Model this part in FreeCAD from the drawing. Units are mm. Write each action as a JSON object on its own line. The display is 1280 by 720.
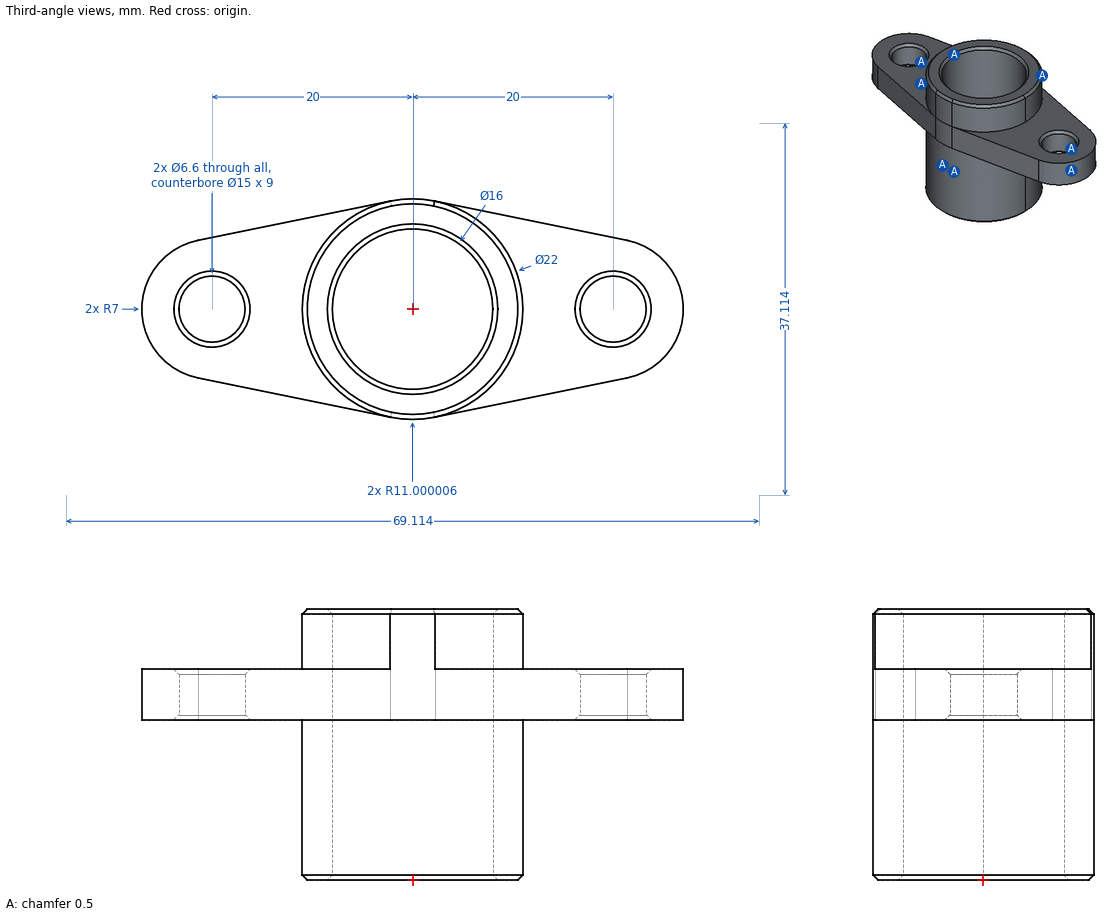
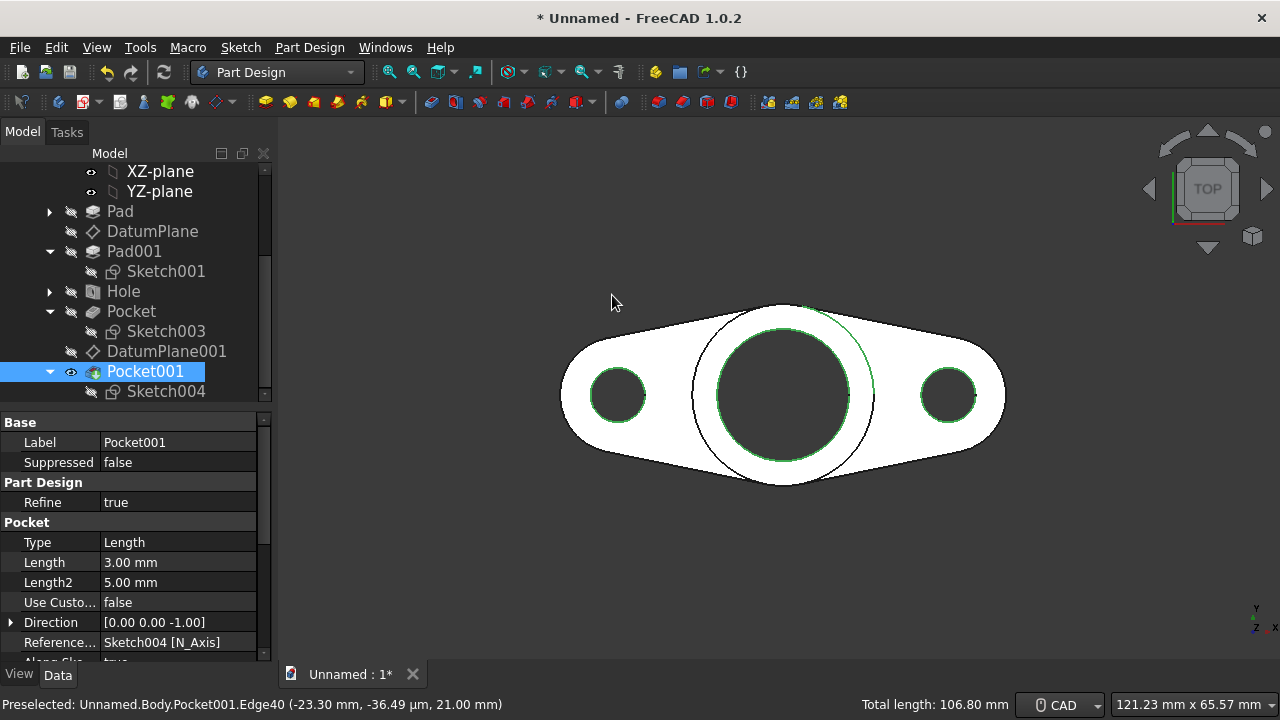
{"action": "left_click", "coordinate": [390, 72]}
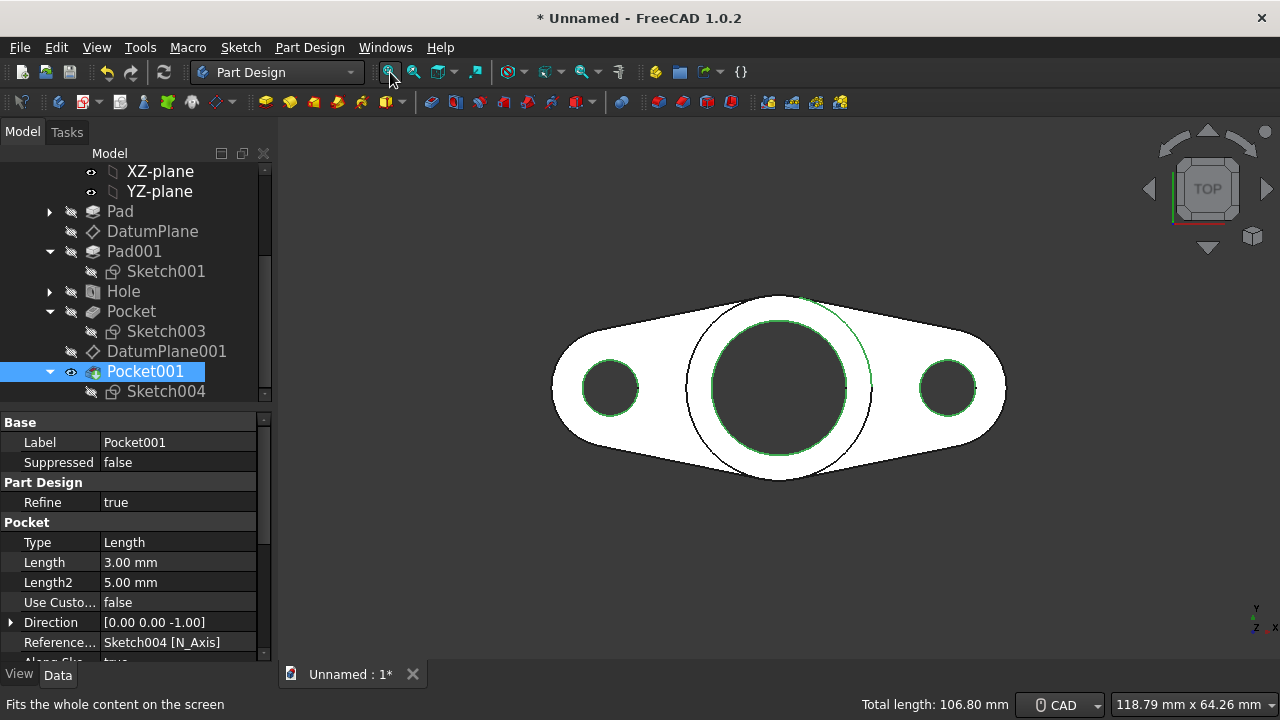
{"action": "key", "text": "1"}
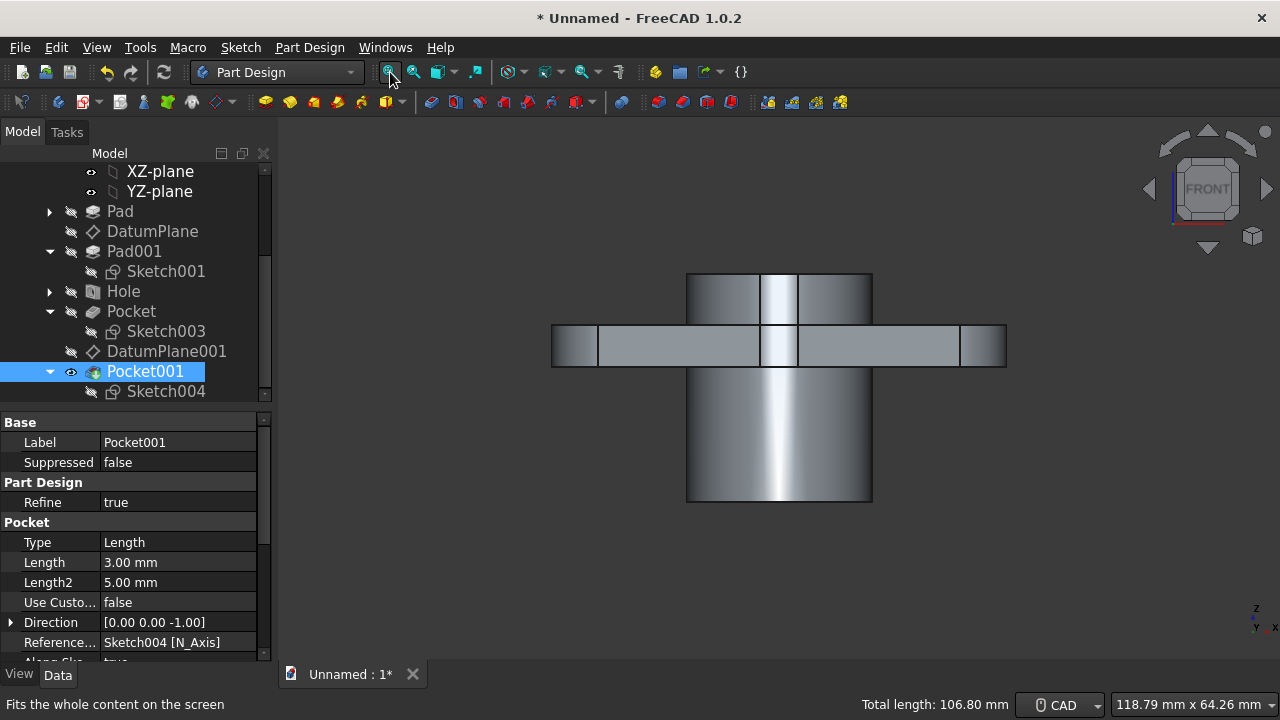
{"action": "left_click", "coordinate": [847, 501], "text": "ctrl"}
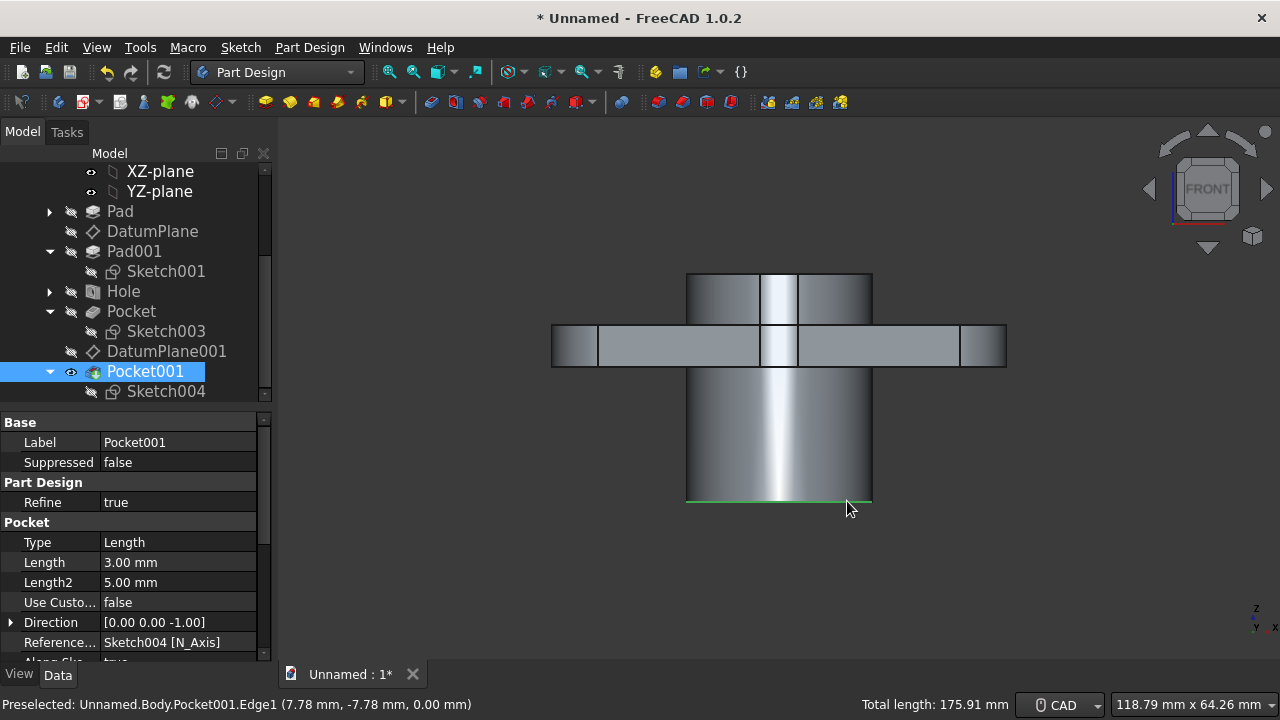
{"action": "key", "text": "3"}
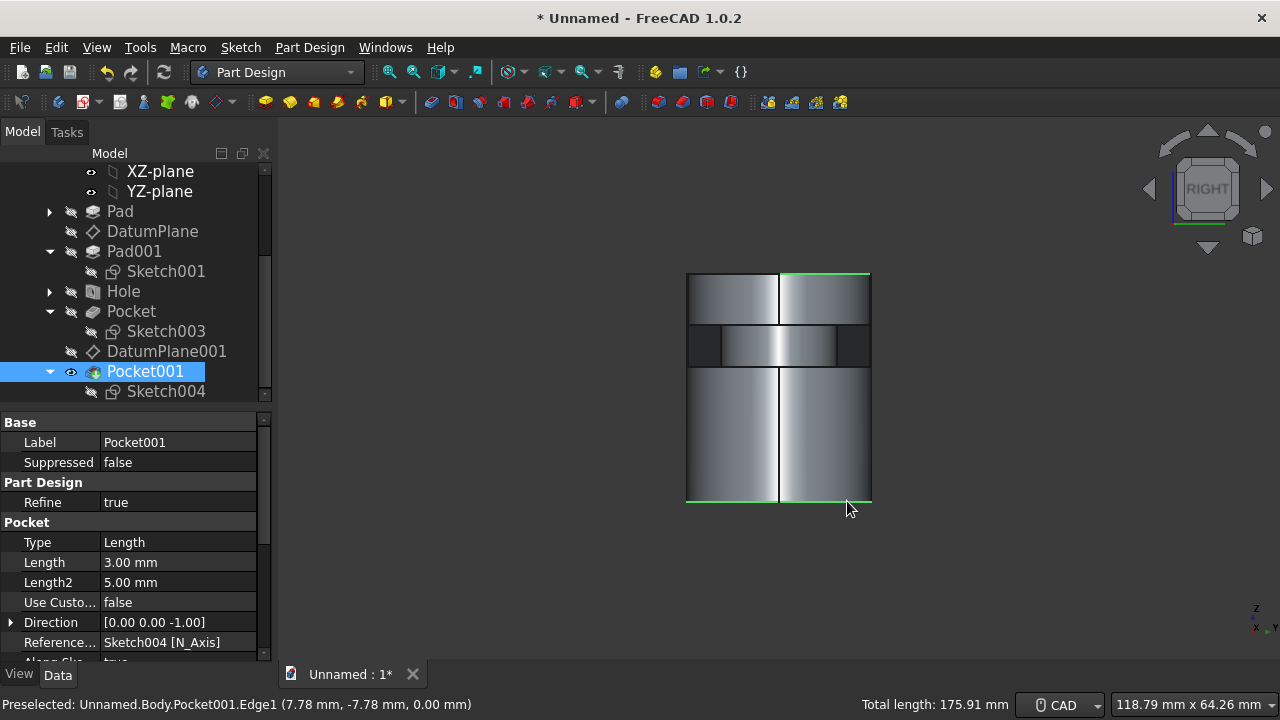
{"action": "left_click", "coordinate": [390, 72]}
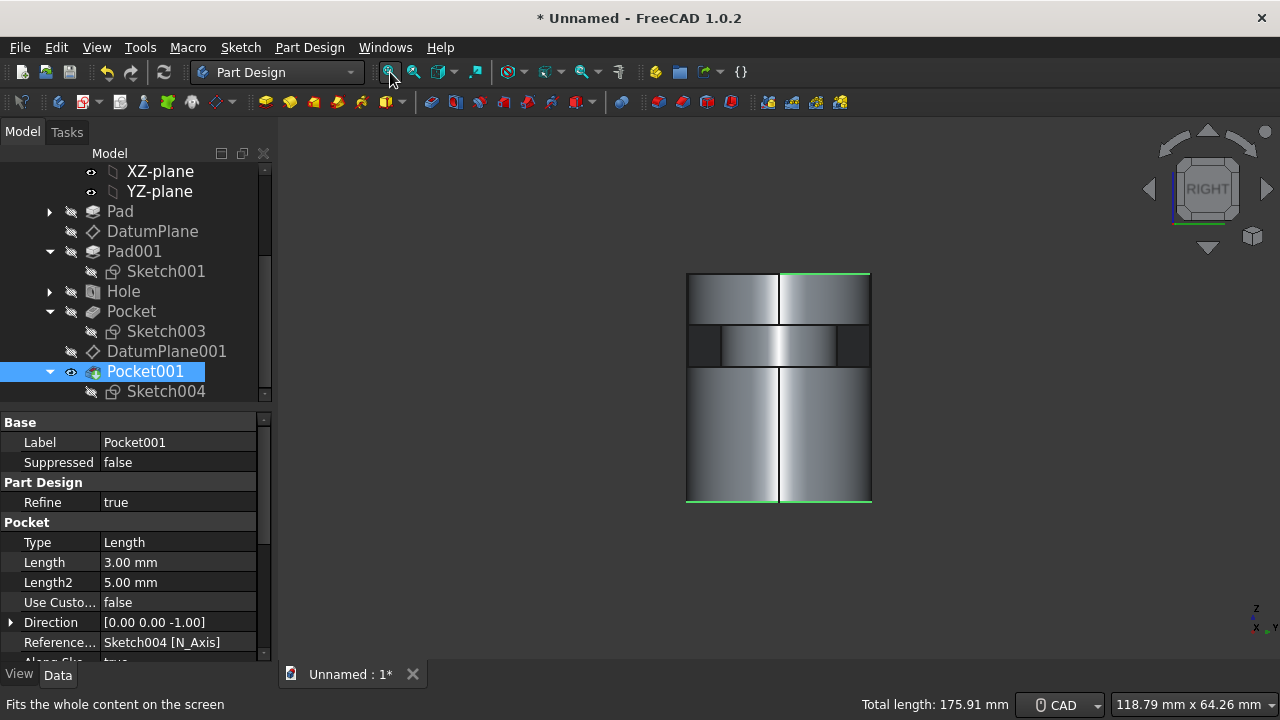
{"action": "key", "text": "5"}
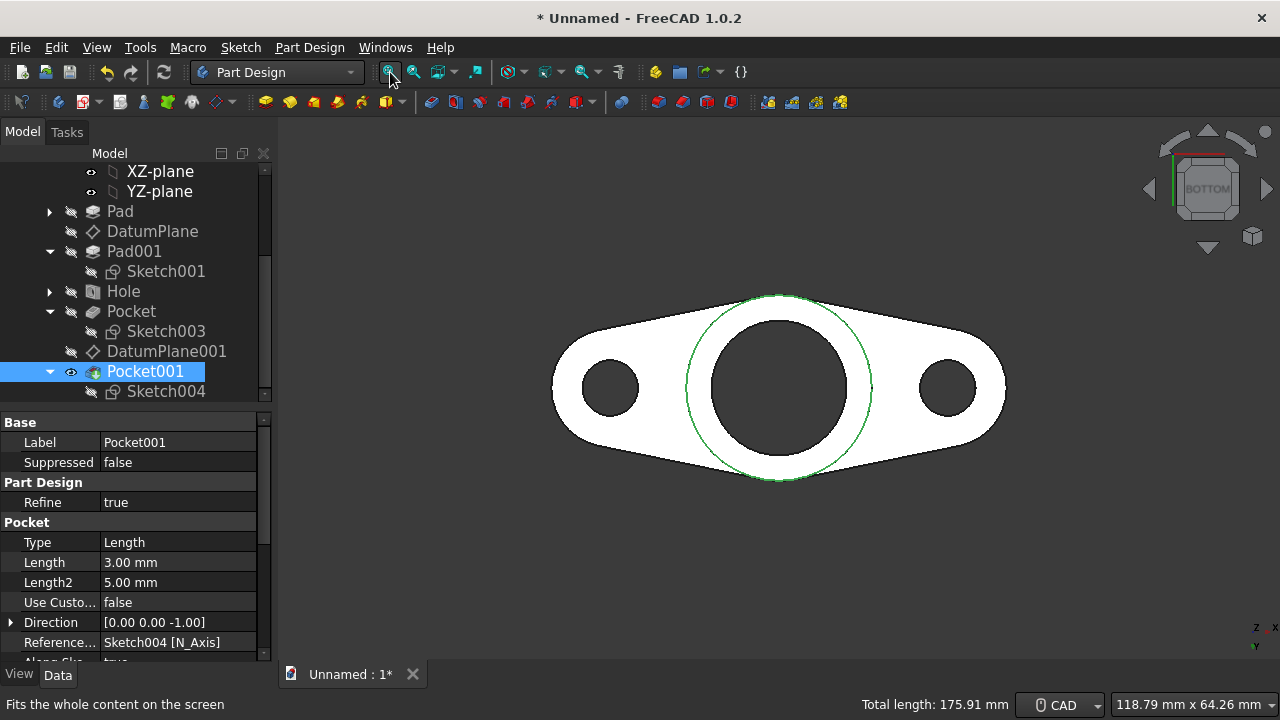
{"action": "left_click", "coordinate": [920, 387], "text": "ctrl"}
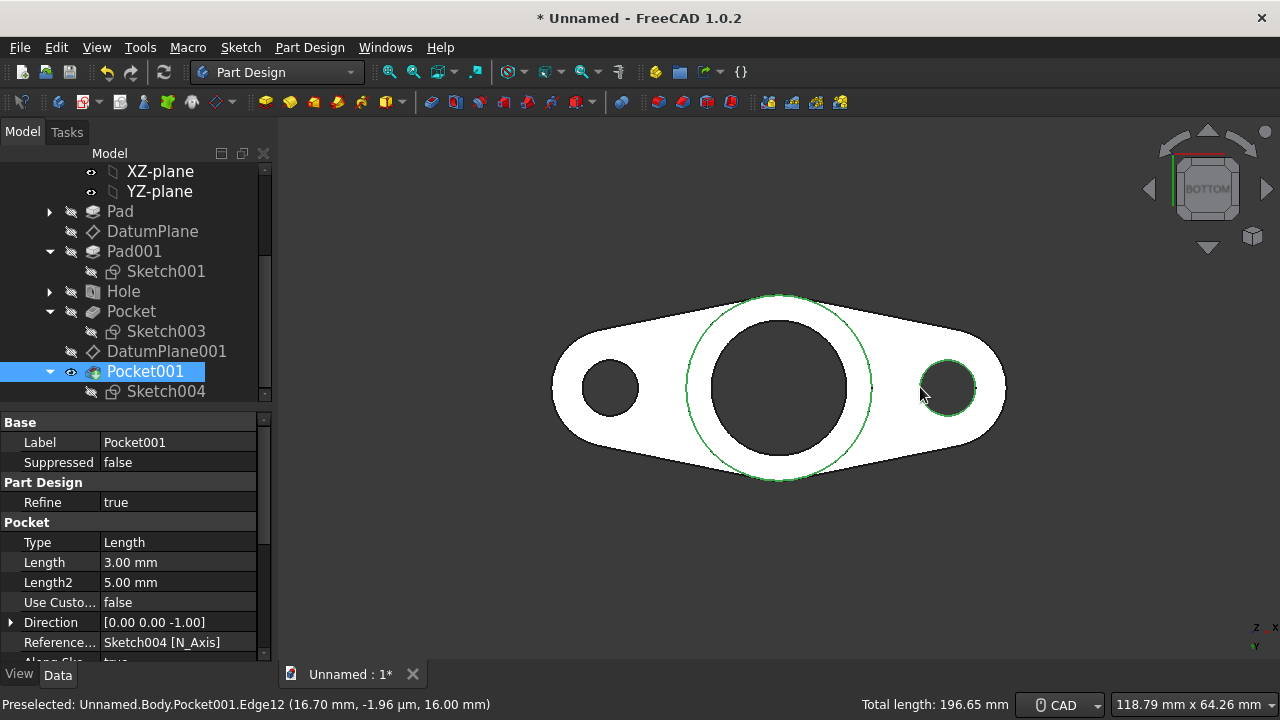
{"action": "left_click", "coordinate": [758, 451], "text": "ctrl"}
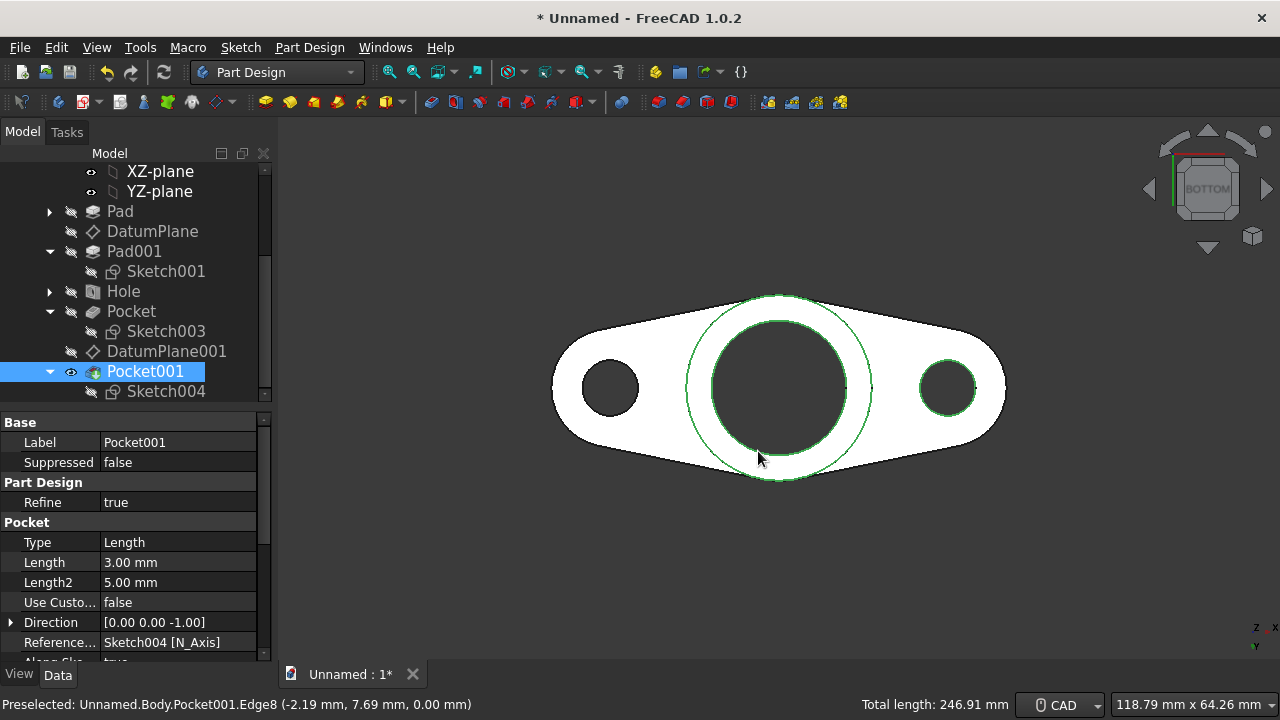
{"action": "left_click", "coordinate": [582, 387], "text": "ctrl"}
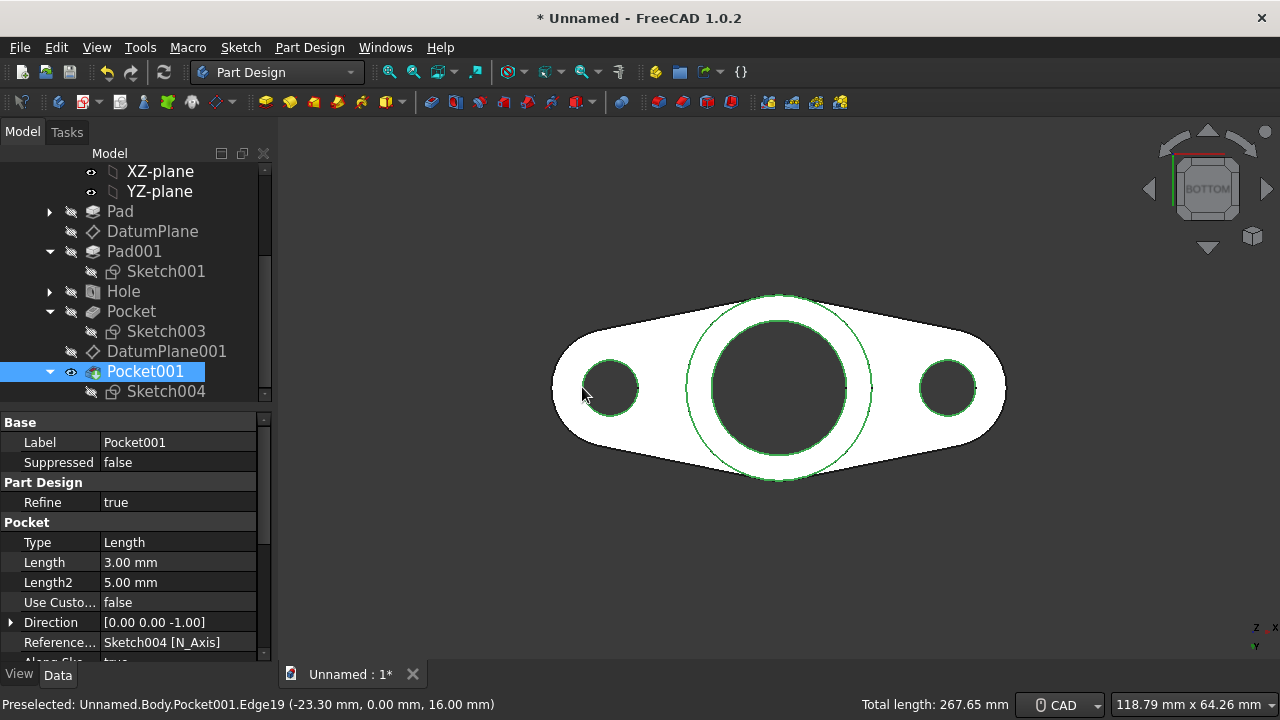
{"action": "left_click", "coordinate": [684, 102]}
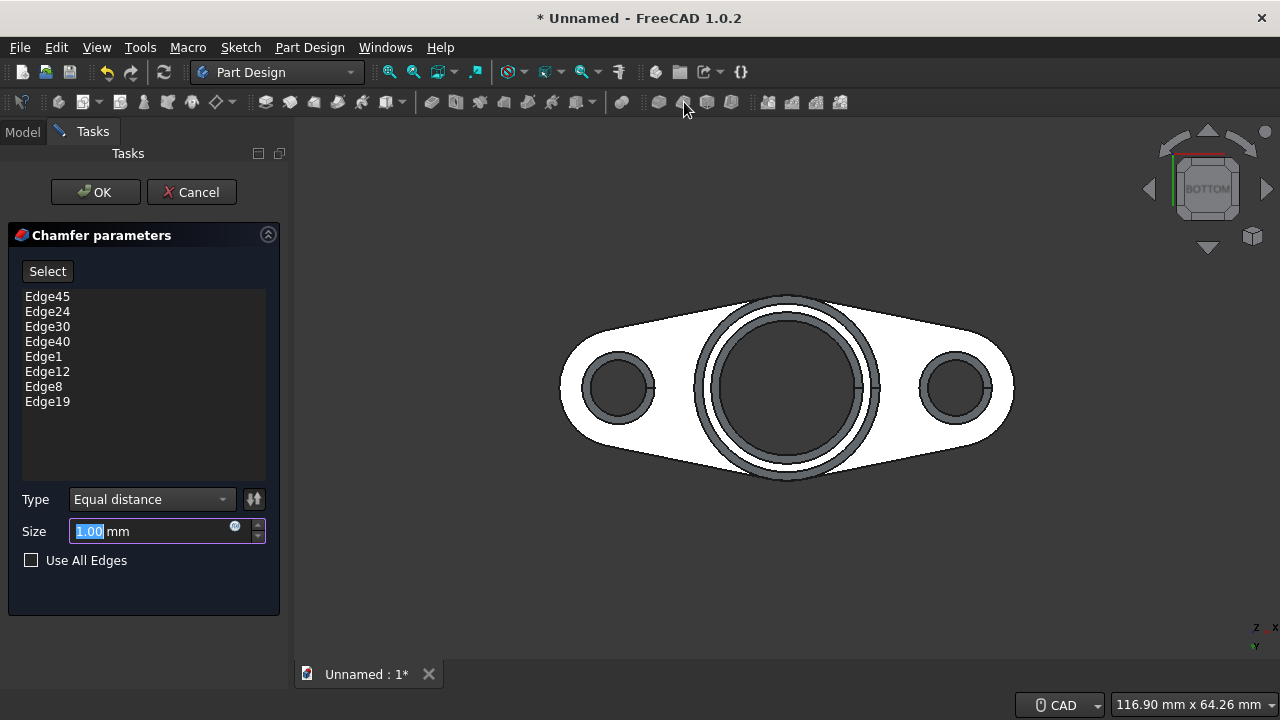
{"action": "type", "text": "0.5"}
{"action": "key", "text": "Tab"}